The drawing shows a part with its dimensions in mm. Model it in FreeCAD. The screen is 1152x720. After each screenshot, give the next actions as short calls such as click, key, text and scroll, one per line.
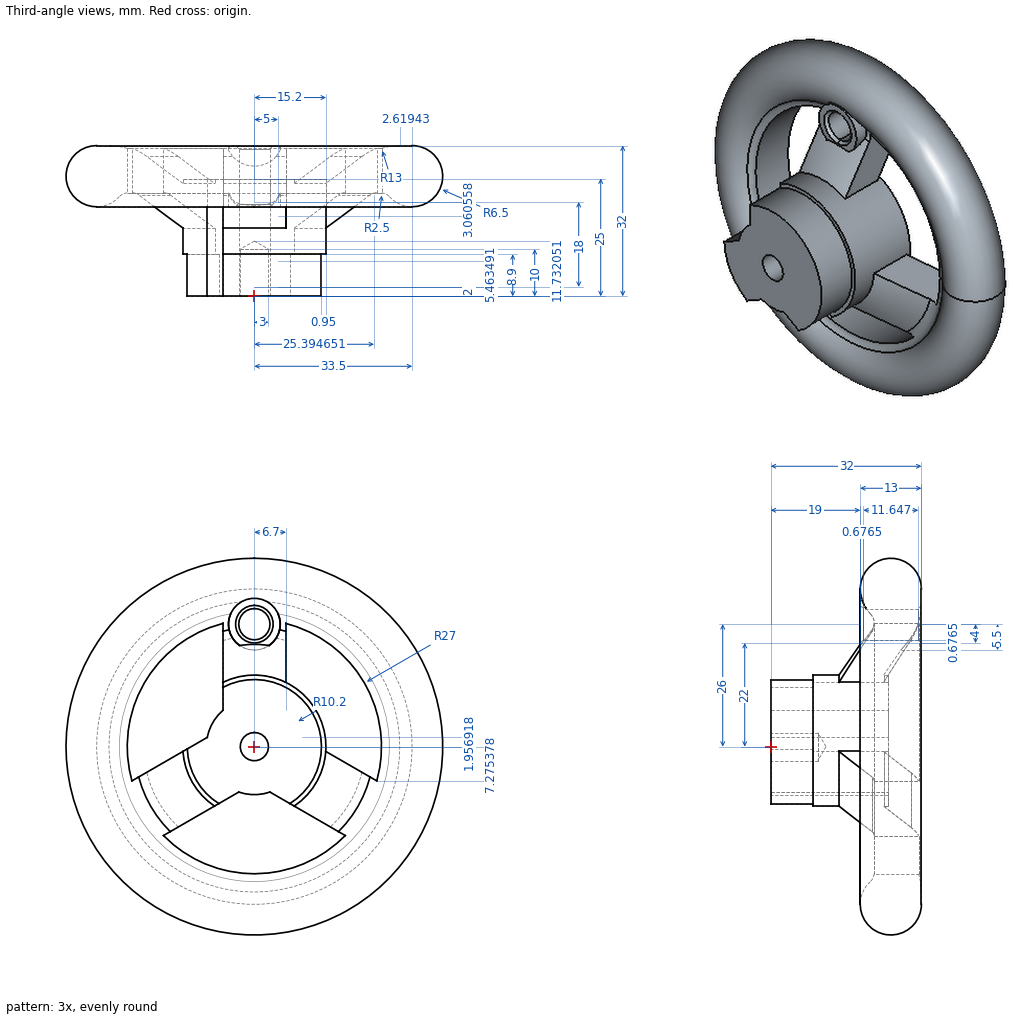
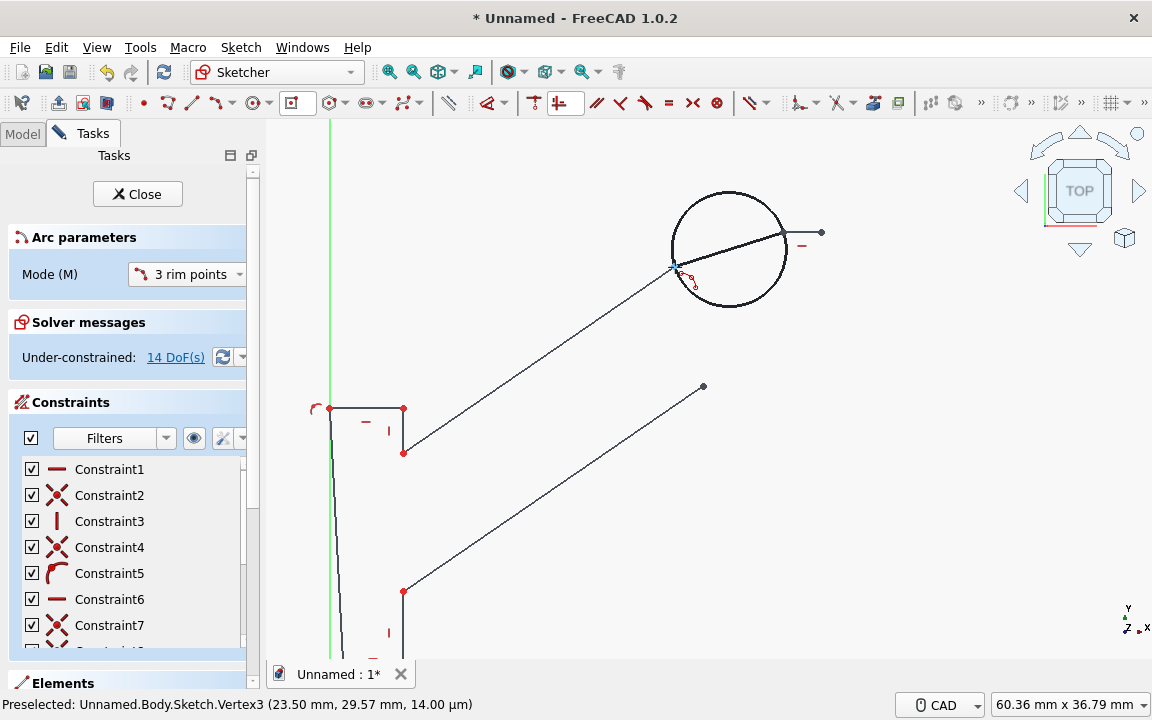
scroll(726, 240, up, 4)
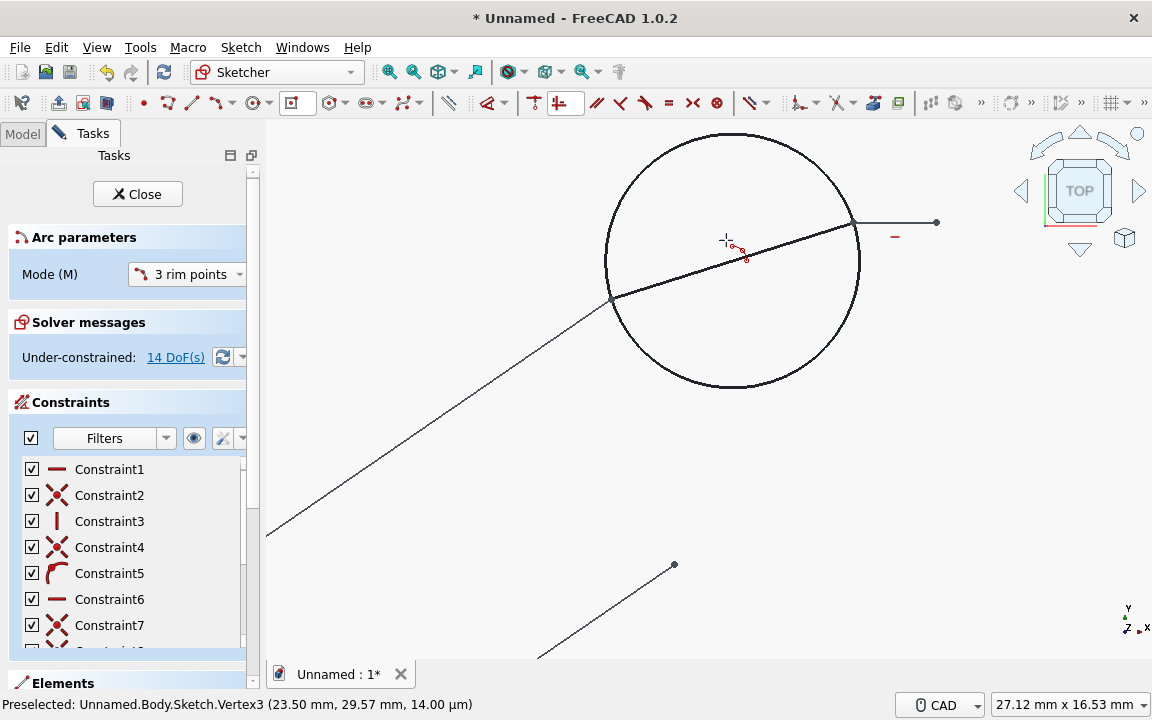
click(726, 239)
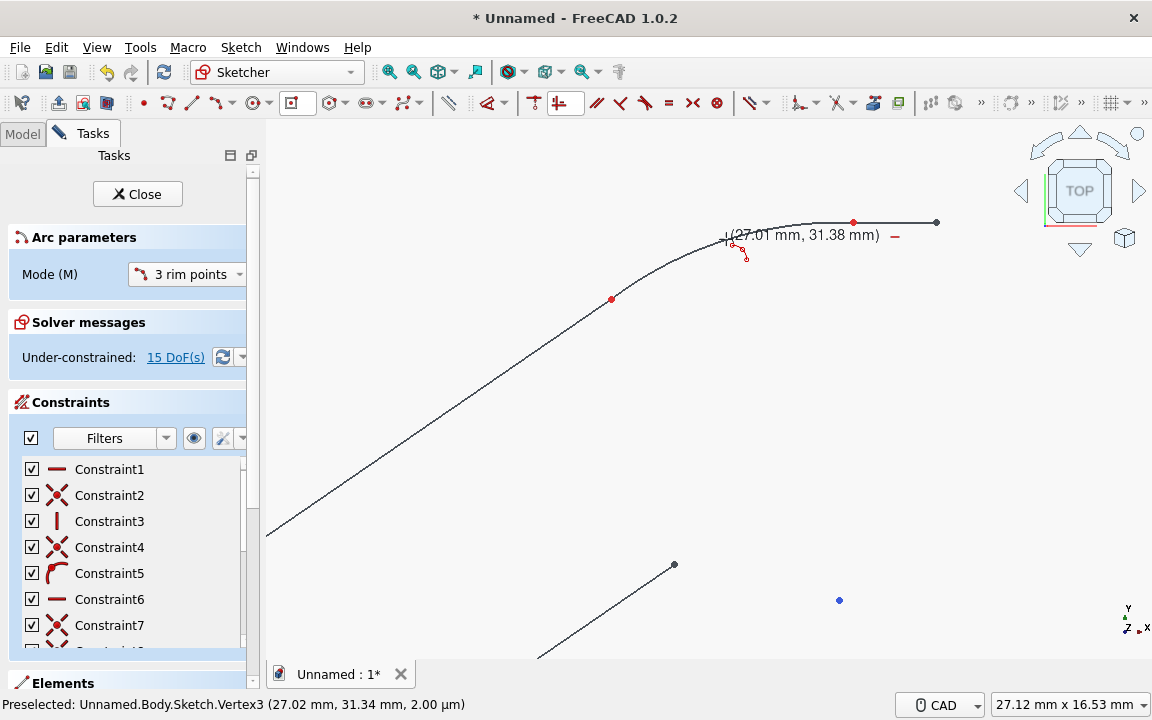
click(675, 565)
click(780, 574)
click(729, 548)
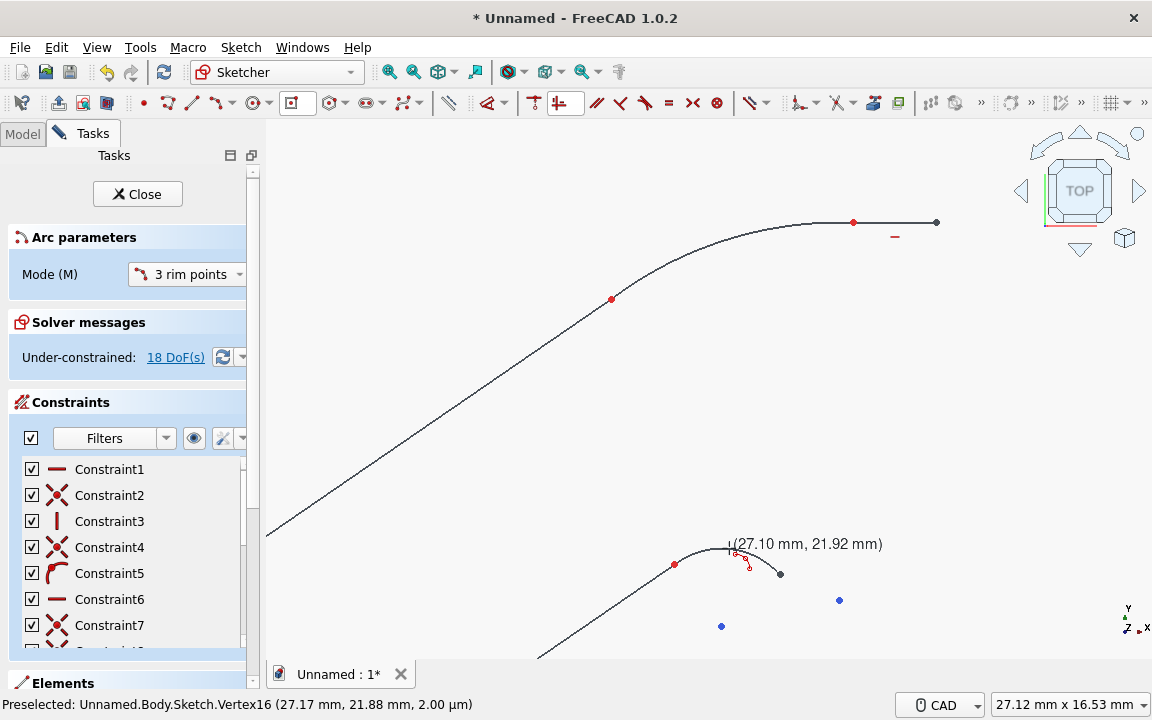
click(780, 575)
click(937, 223)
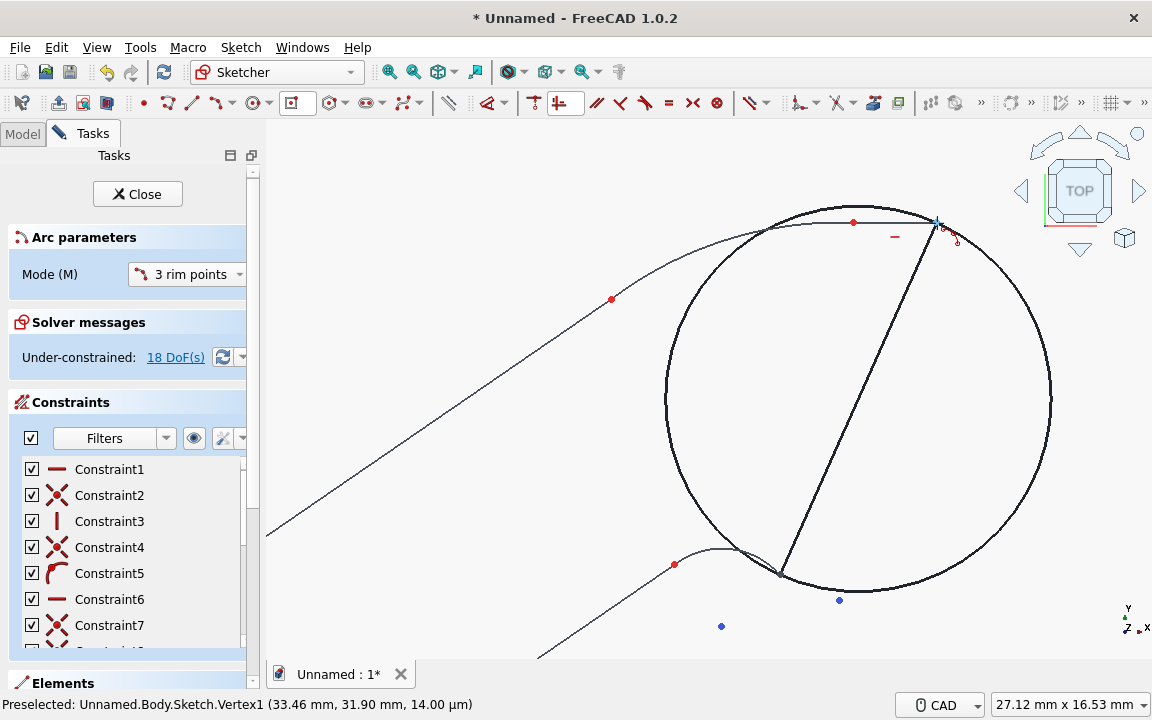
scroll(706, 237, down, 6)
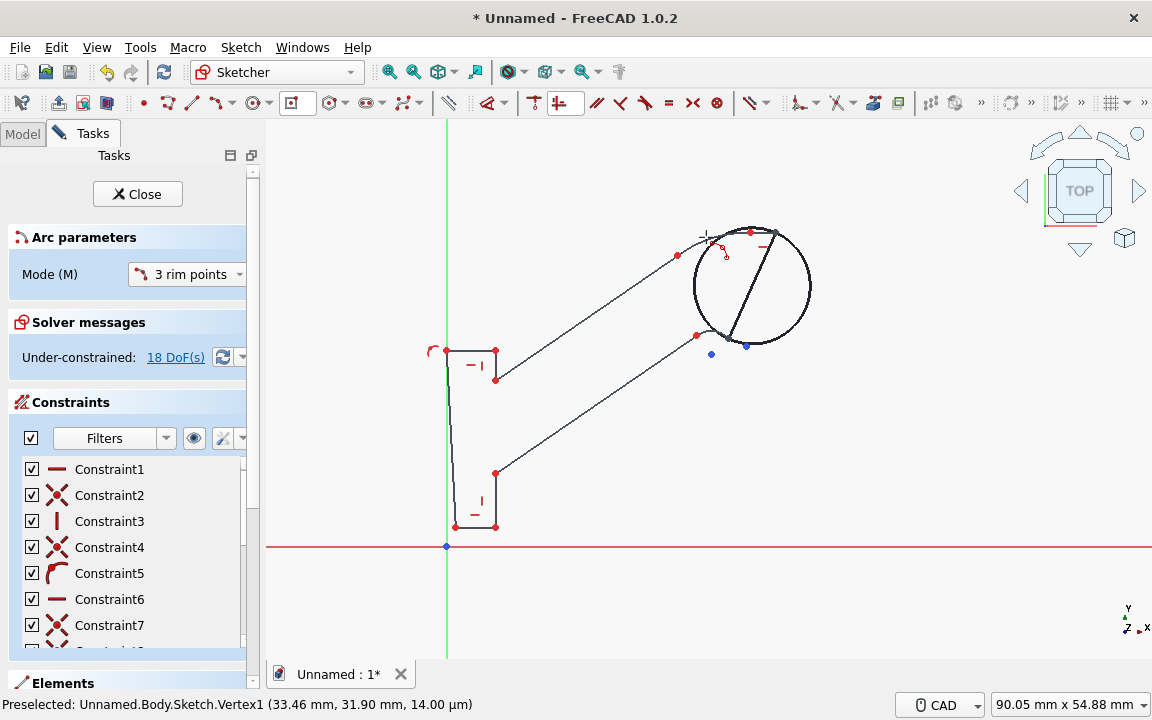
click(835, 322)
key(Escape)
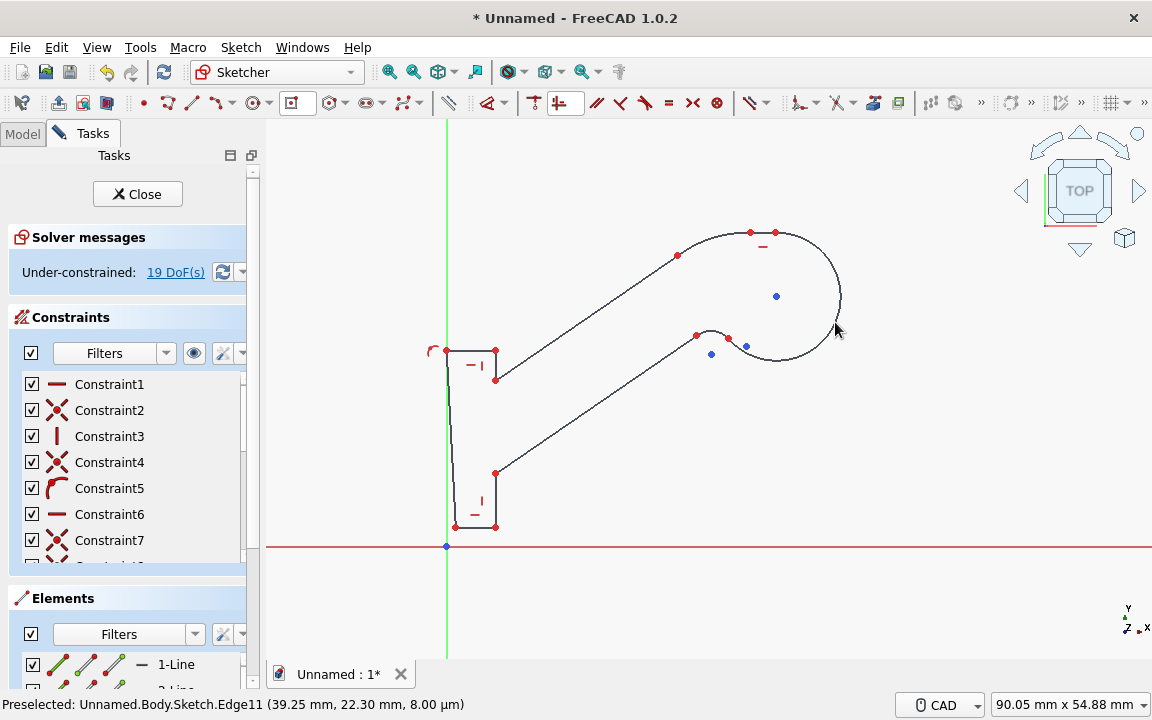
scroll(766, 233, up, 2)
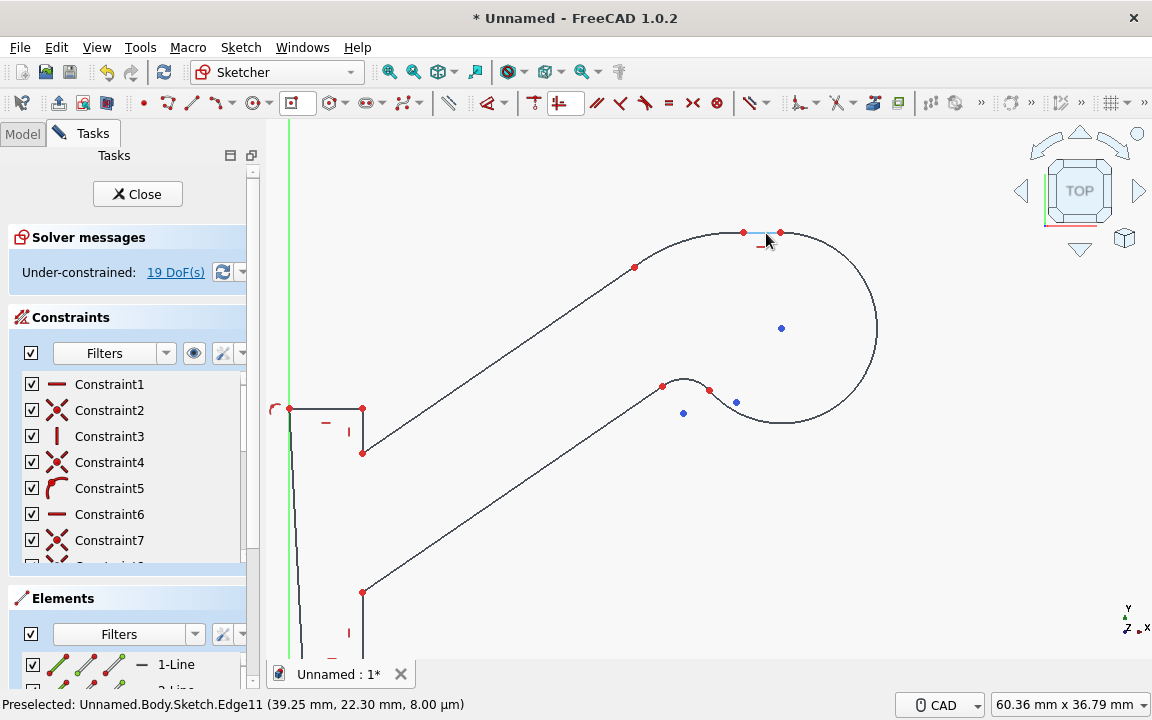
click(766, 233)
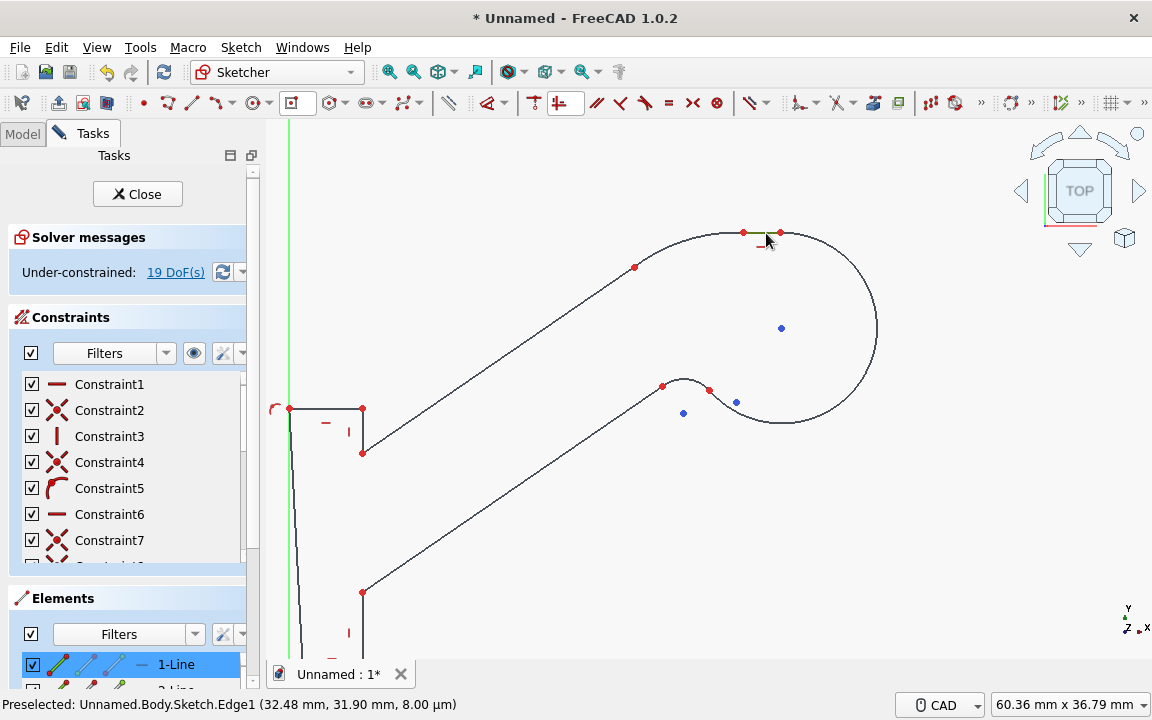
click(708, 235)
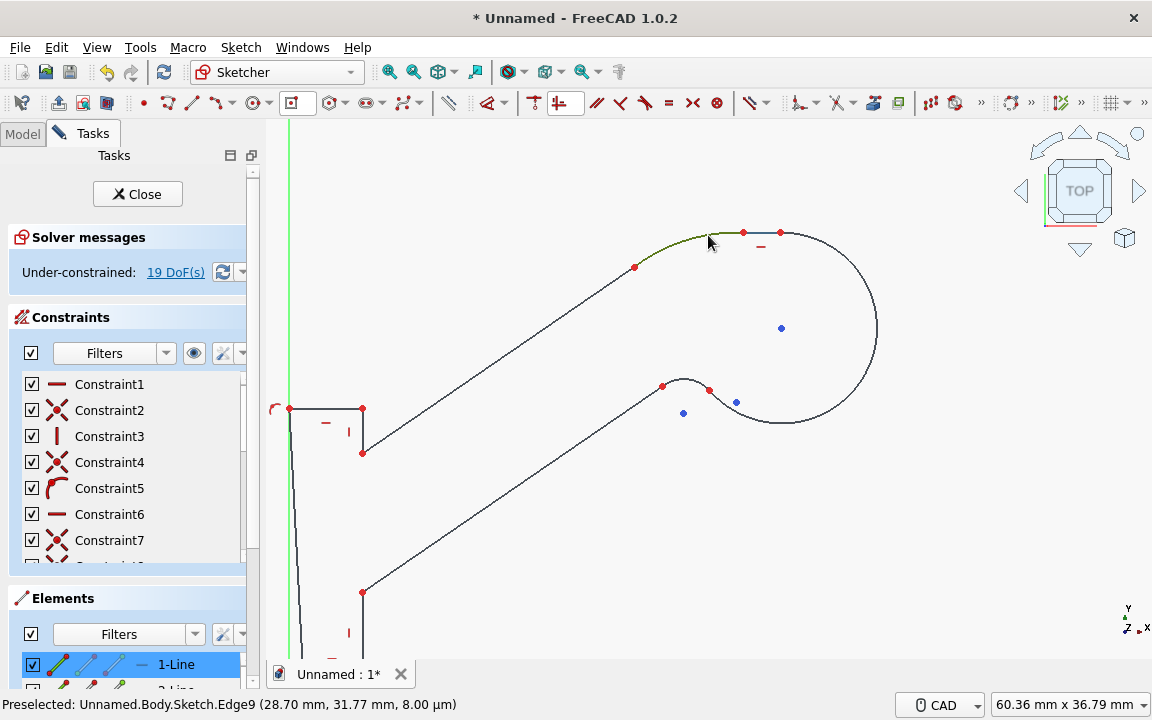
click(646, 104)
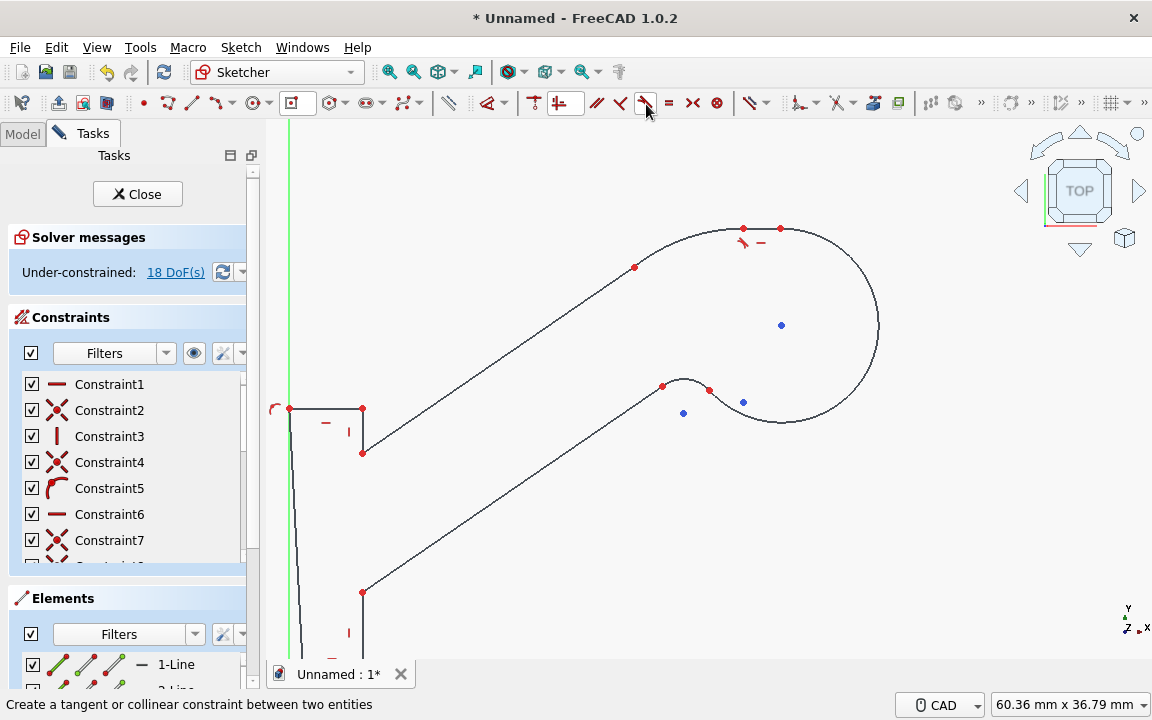
scroll(769, 229, up, 2)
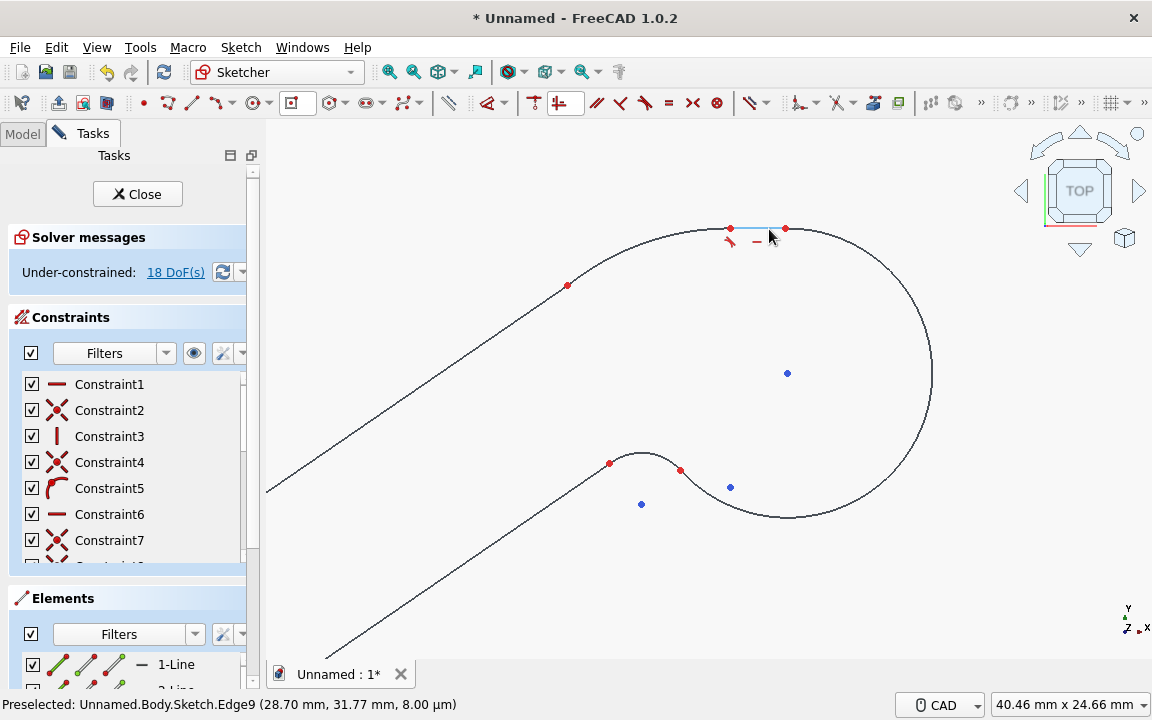
click(769, 228)